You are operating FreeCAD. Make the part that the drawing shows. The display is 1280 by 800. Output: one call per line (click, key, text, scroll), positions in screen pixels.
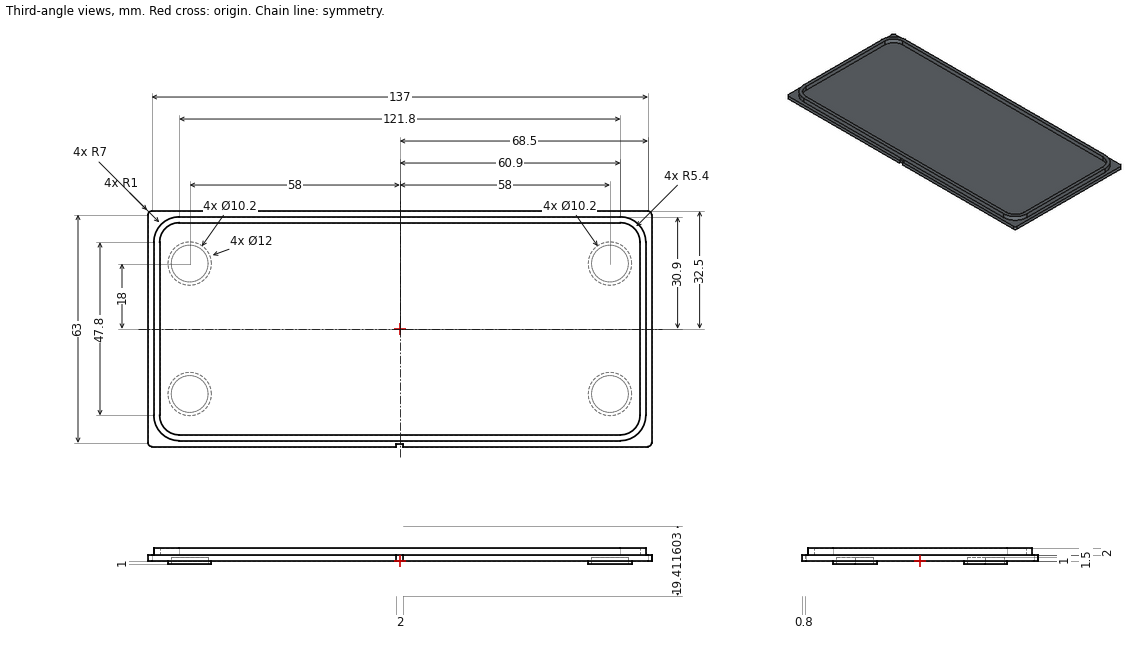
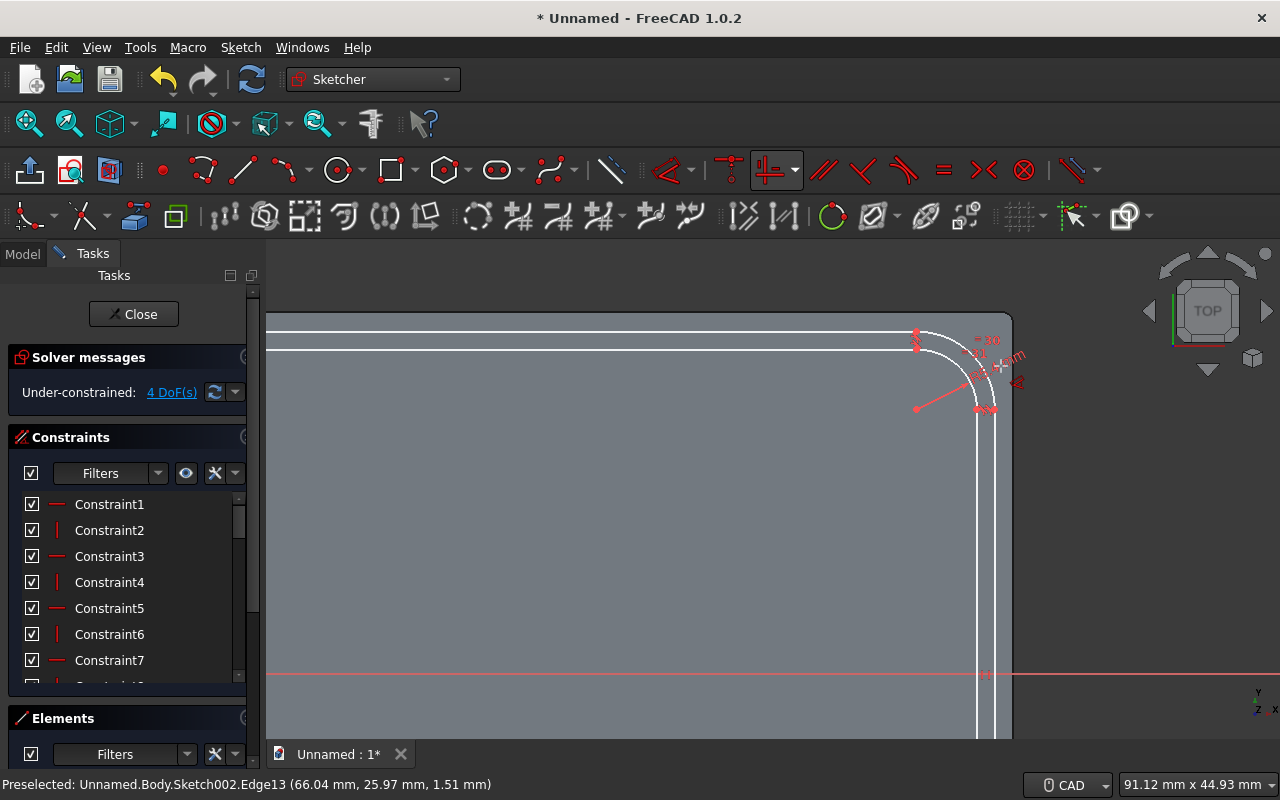
scroll(975, 382, down, 5)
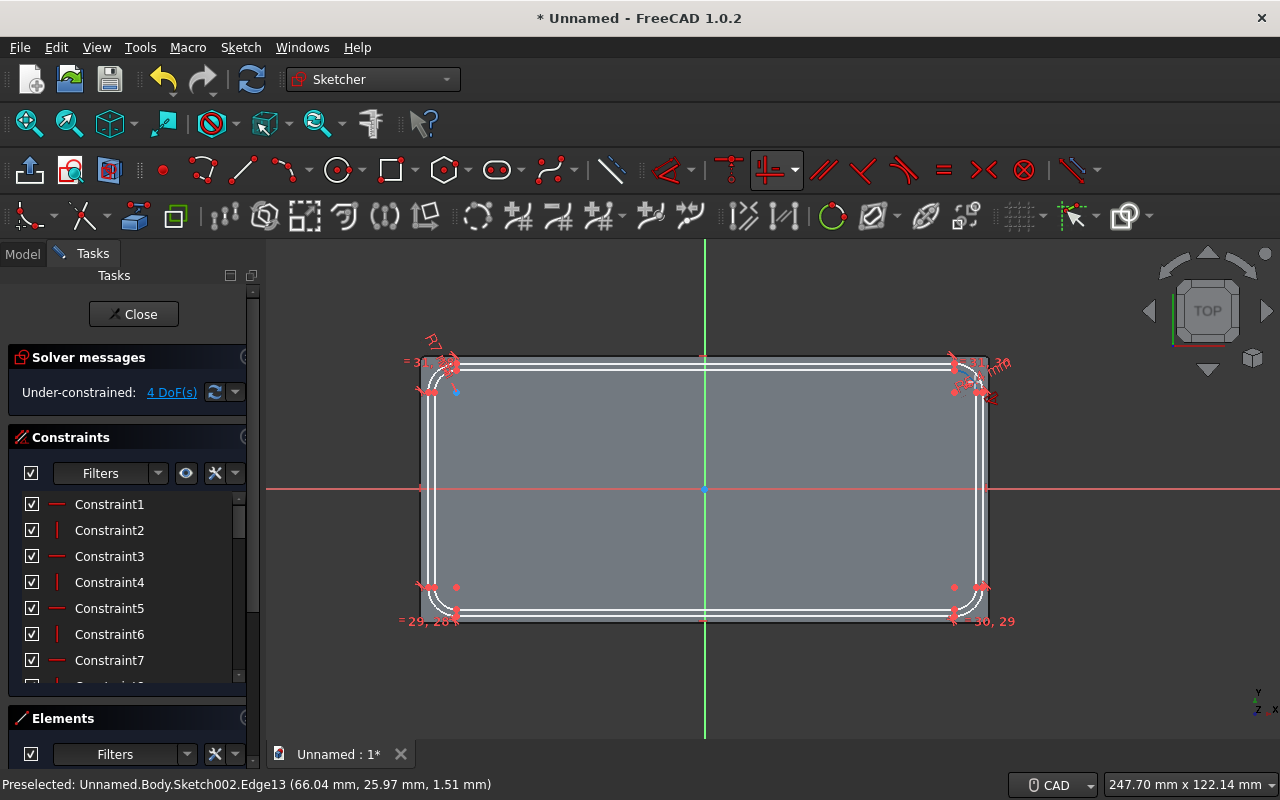
scroll(428, 451, up, 4)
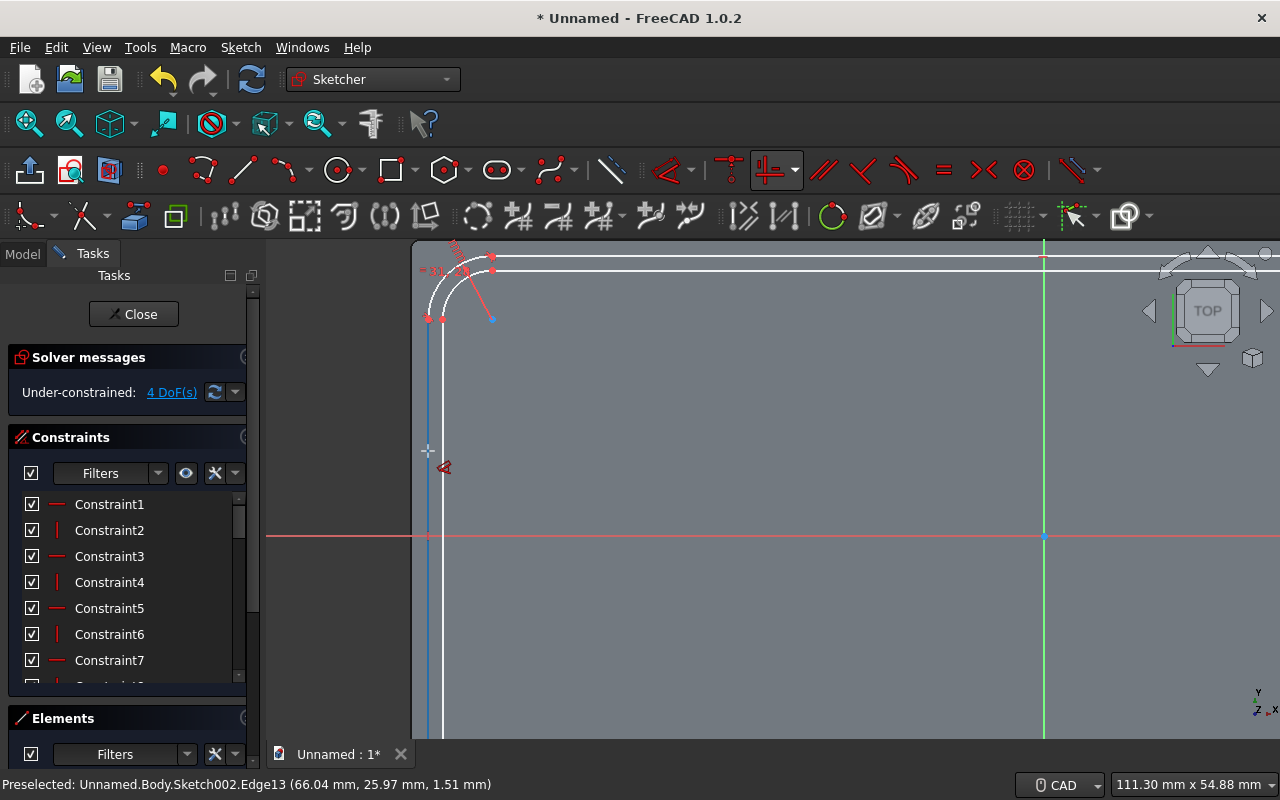
click(428, 450)
click(394, 515)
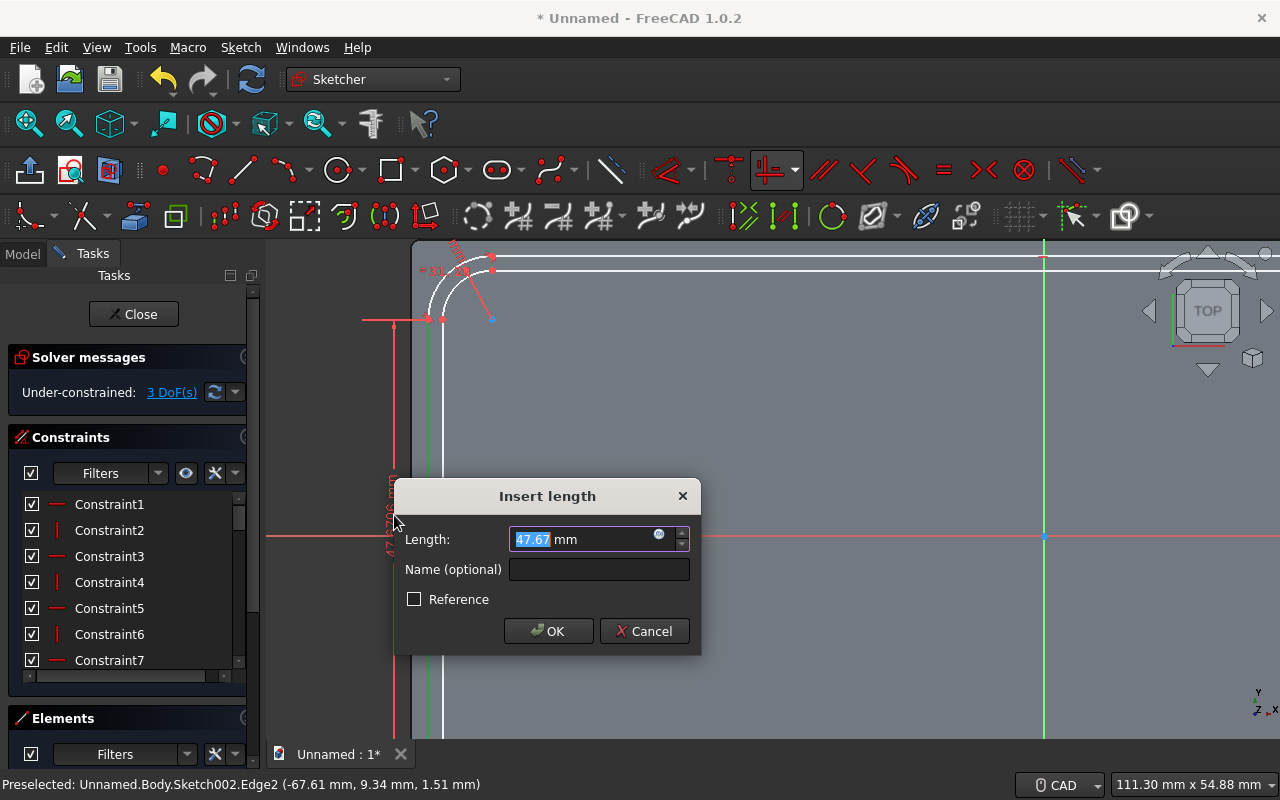
text(47.8)
key(Return)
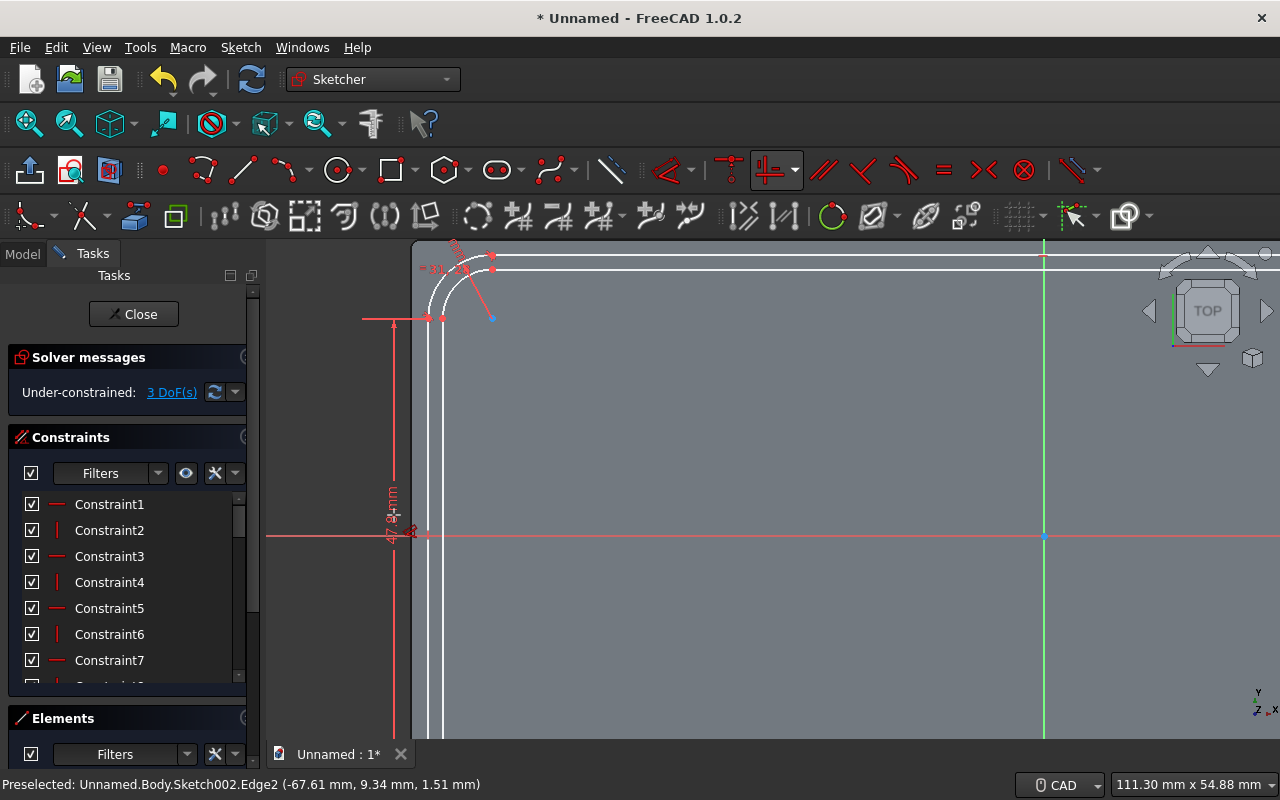
scroll(427, 451, down, 4)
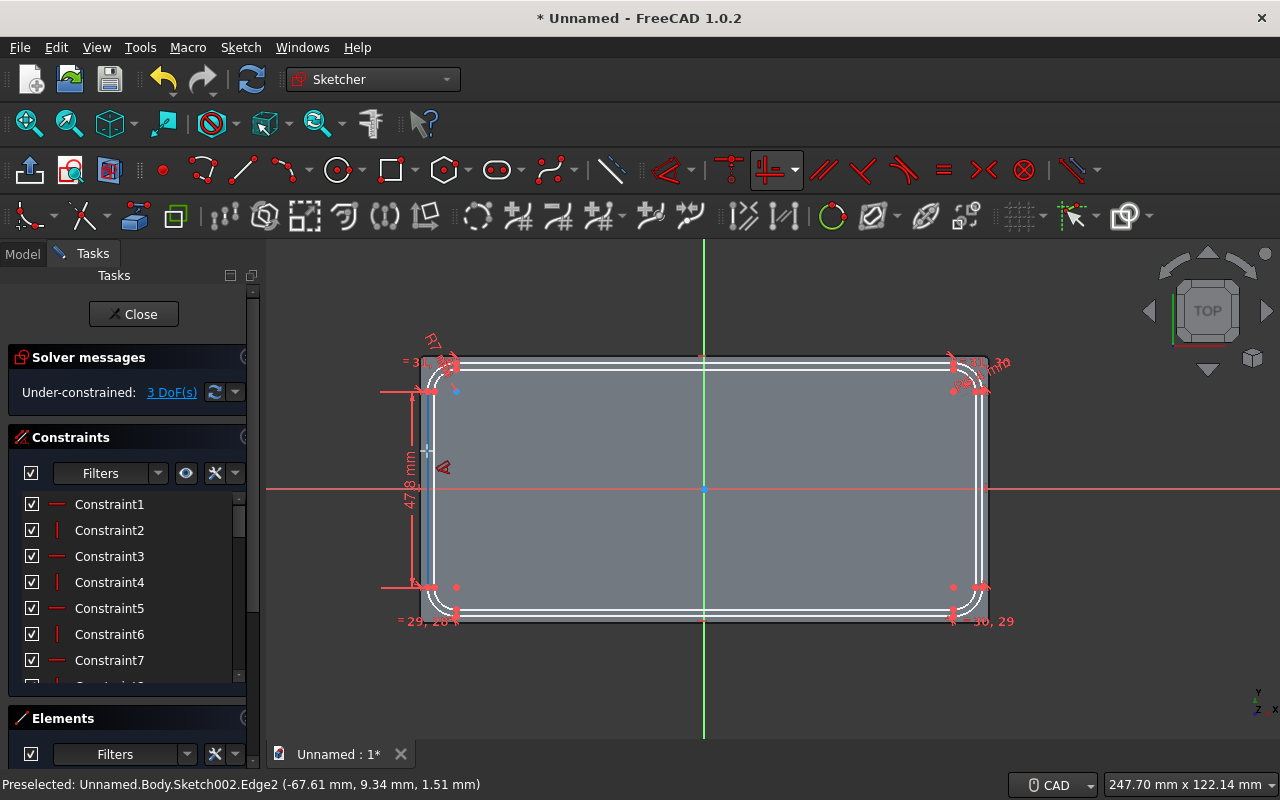
scroll(804, 363, up, 4)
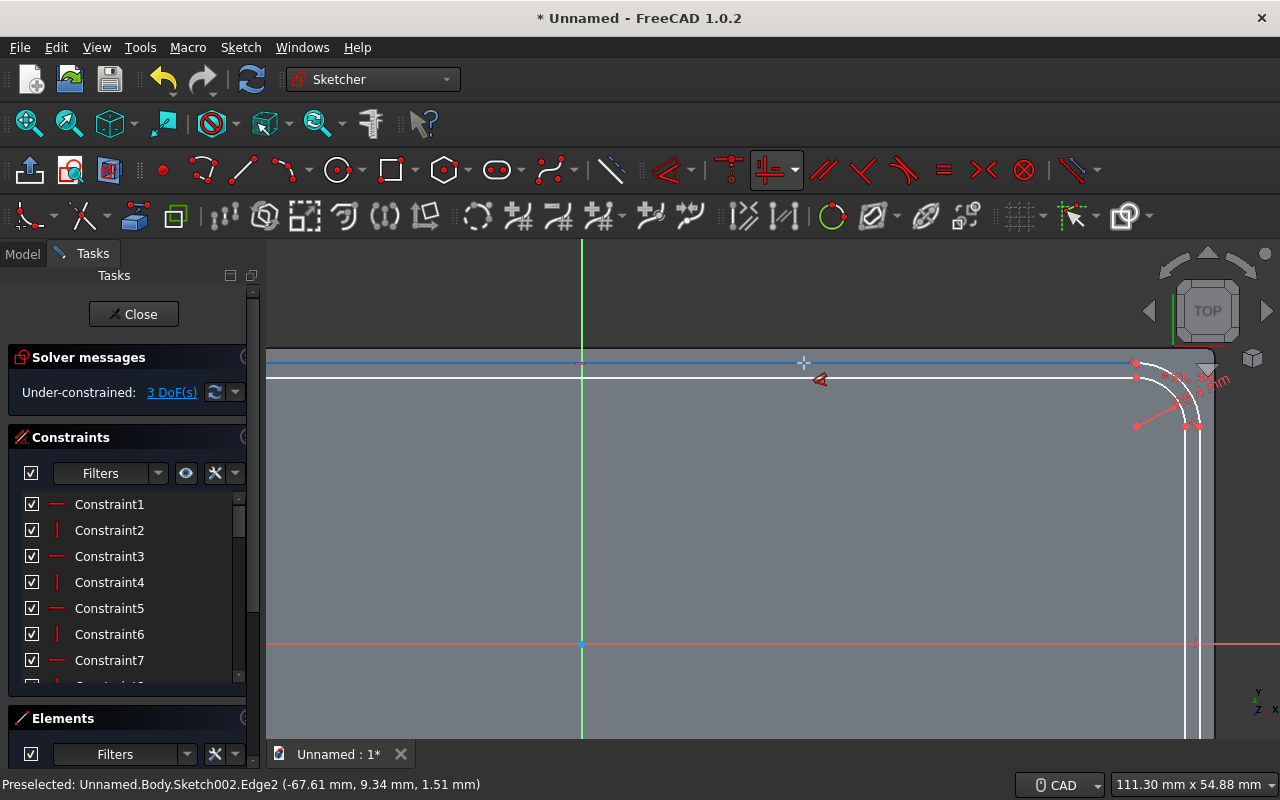
click(804, 363)
click(704, 329)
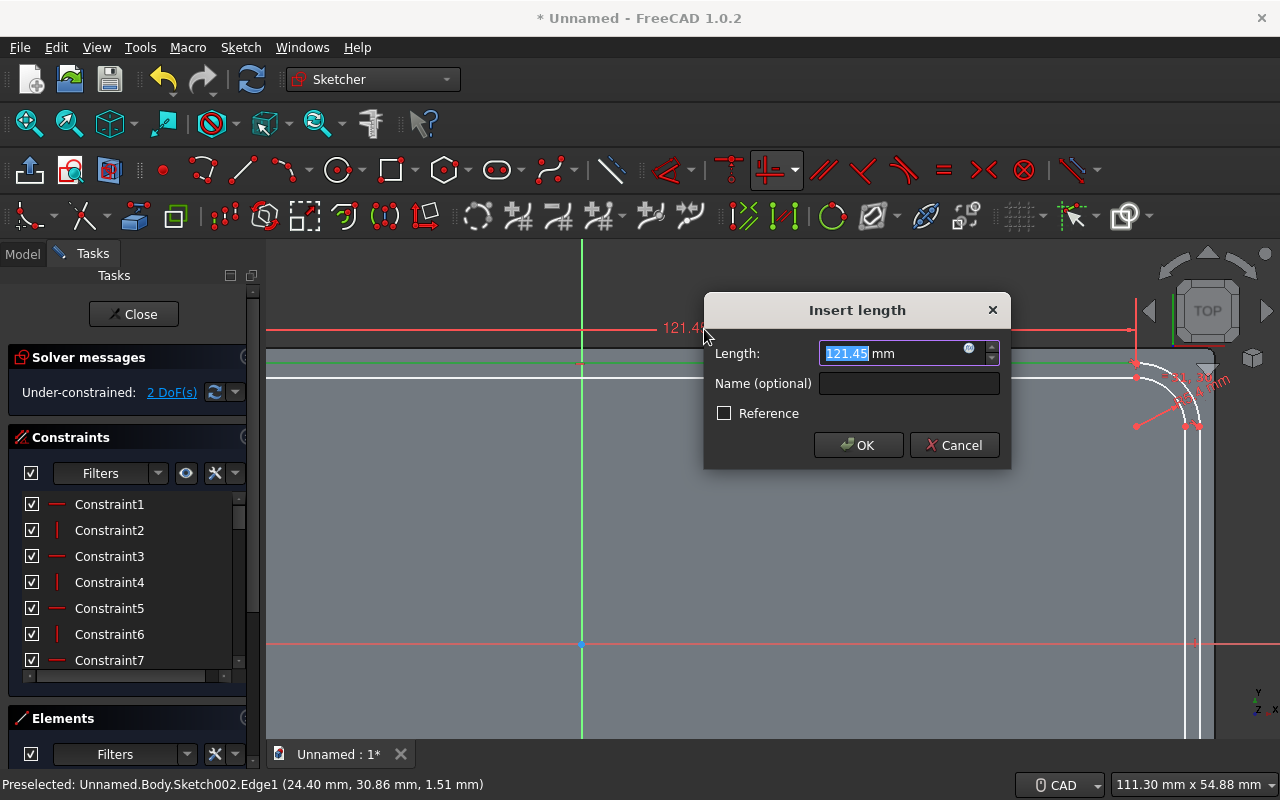
text(121.8)
key(Return)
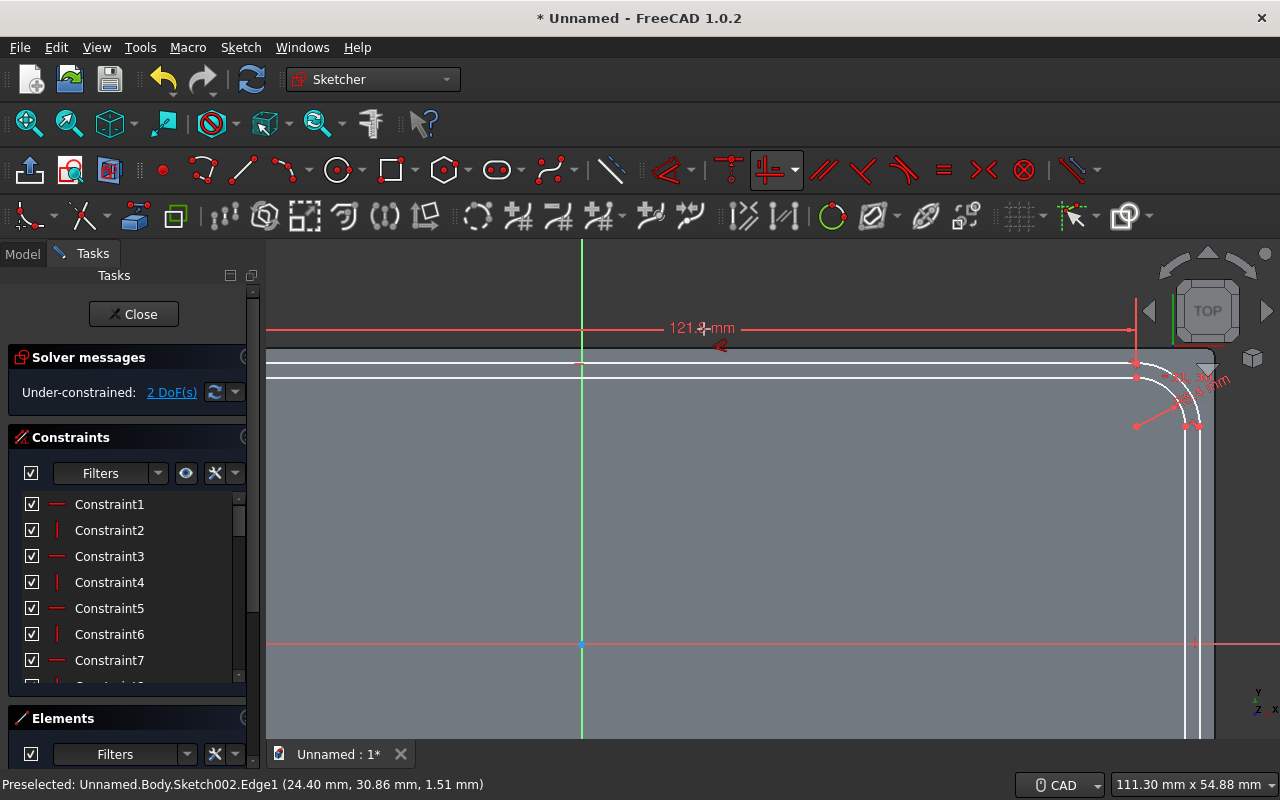
scroll(805, 362, down, 4)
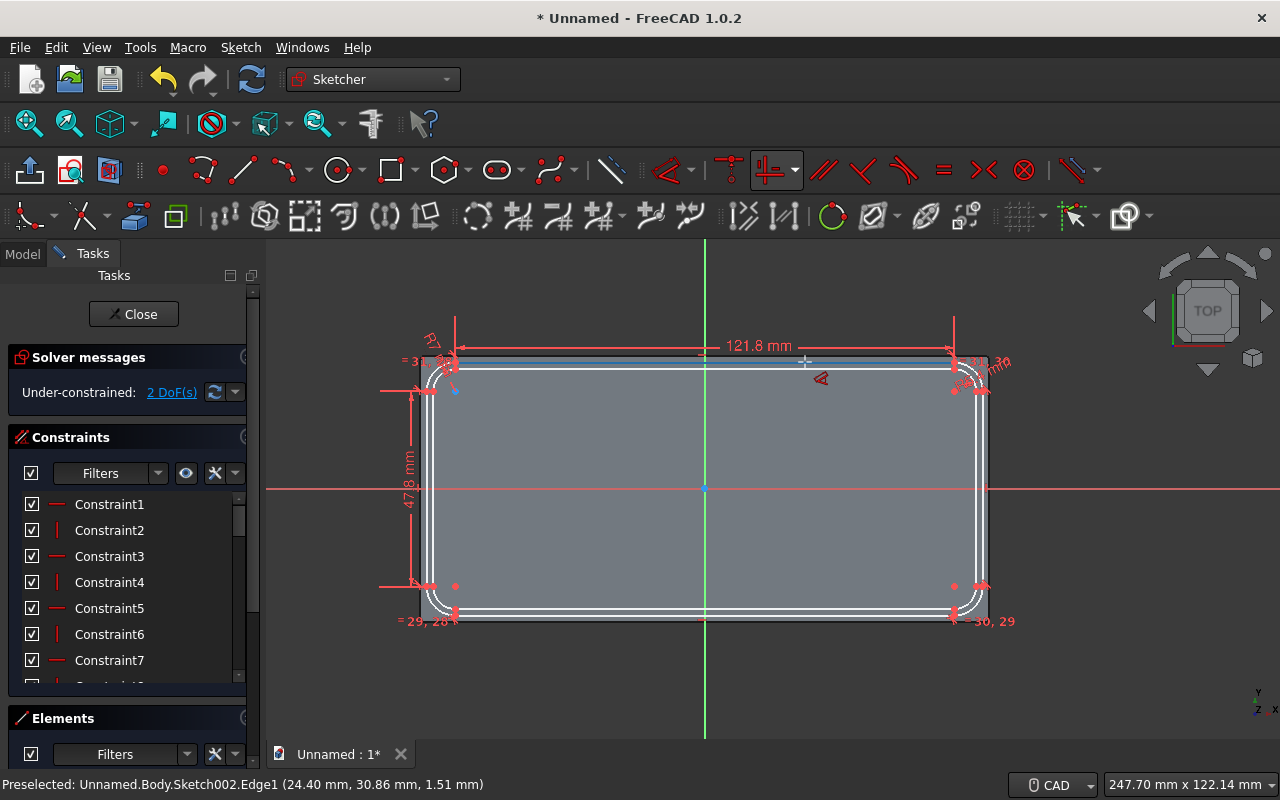
scroll(954, 363, up, 4)